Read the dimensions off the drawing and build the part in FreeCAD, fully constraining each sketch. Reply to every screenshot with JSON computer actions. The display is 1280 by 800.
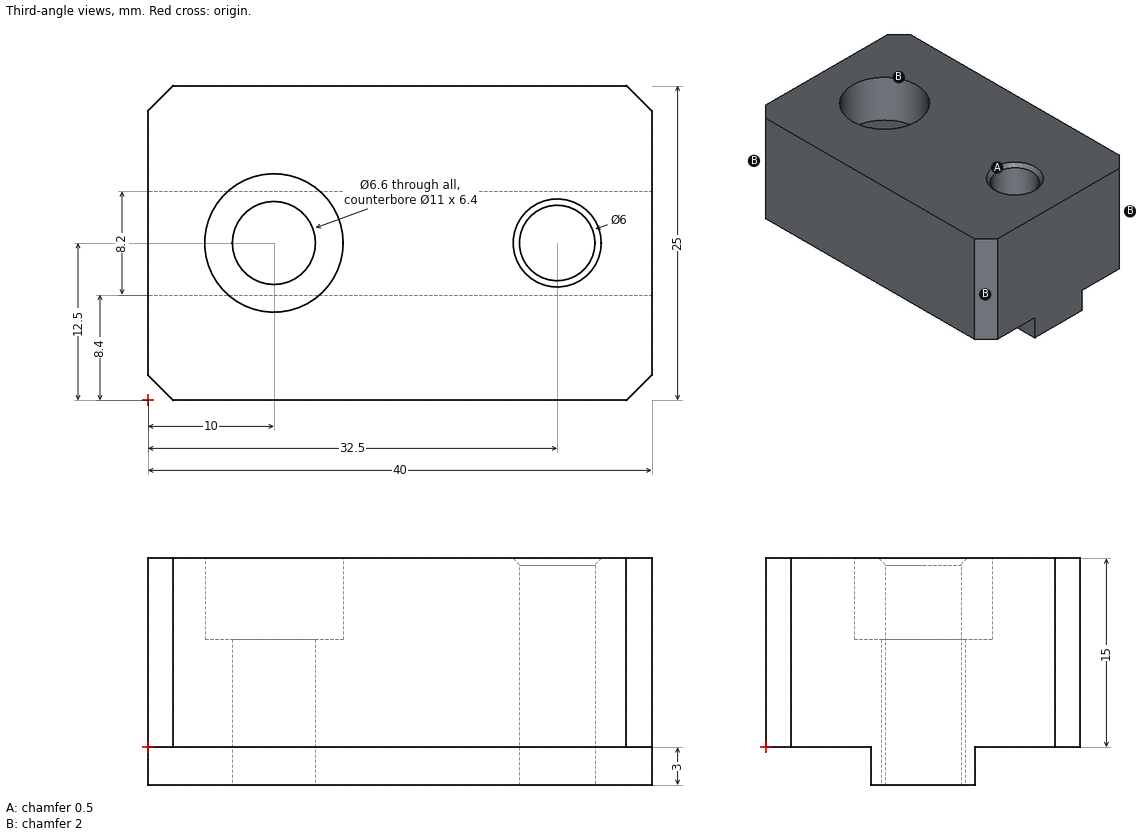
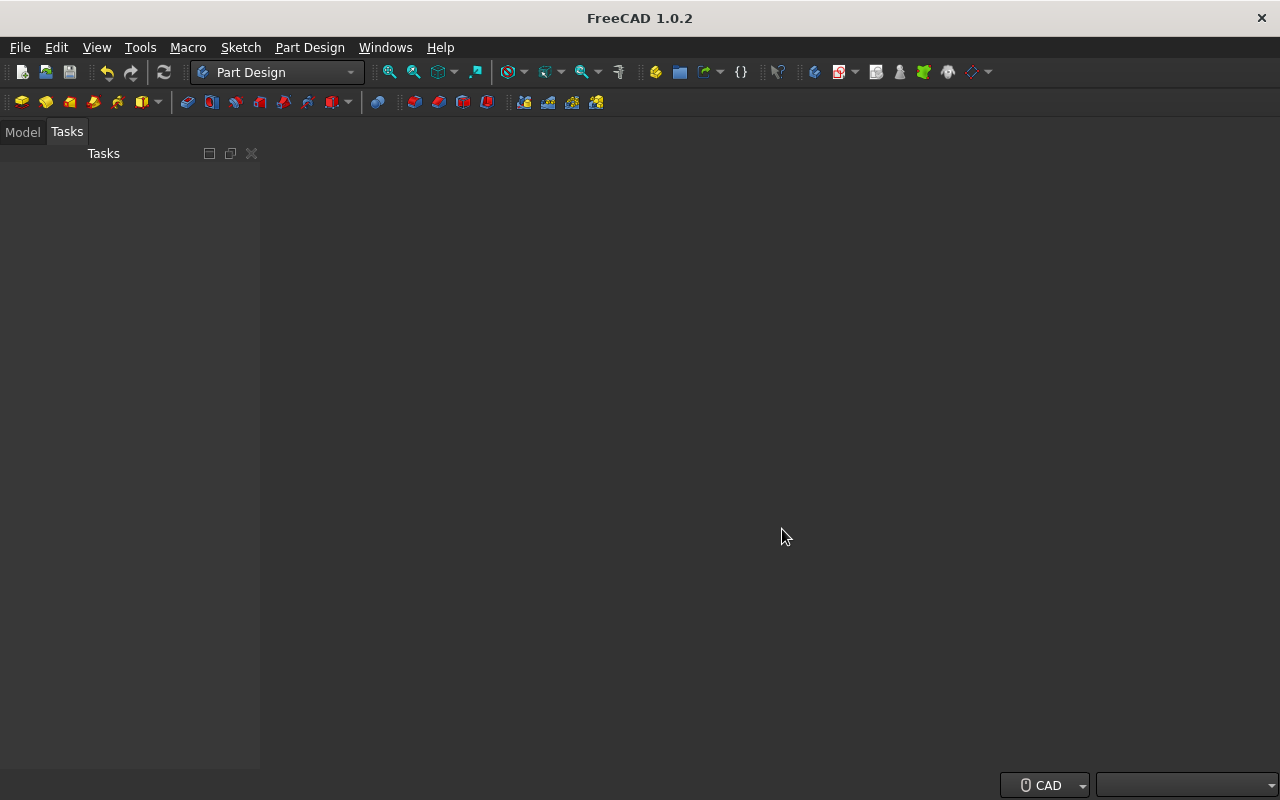
{"action": "left_click", "coordinate": [22, 72]}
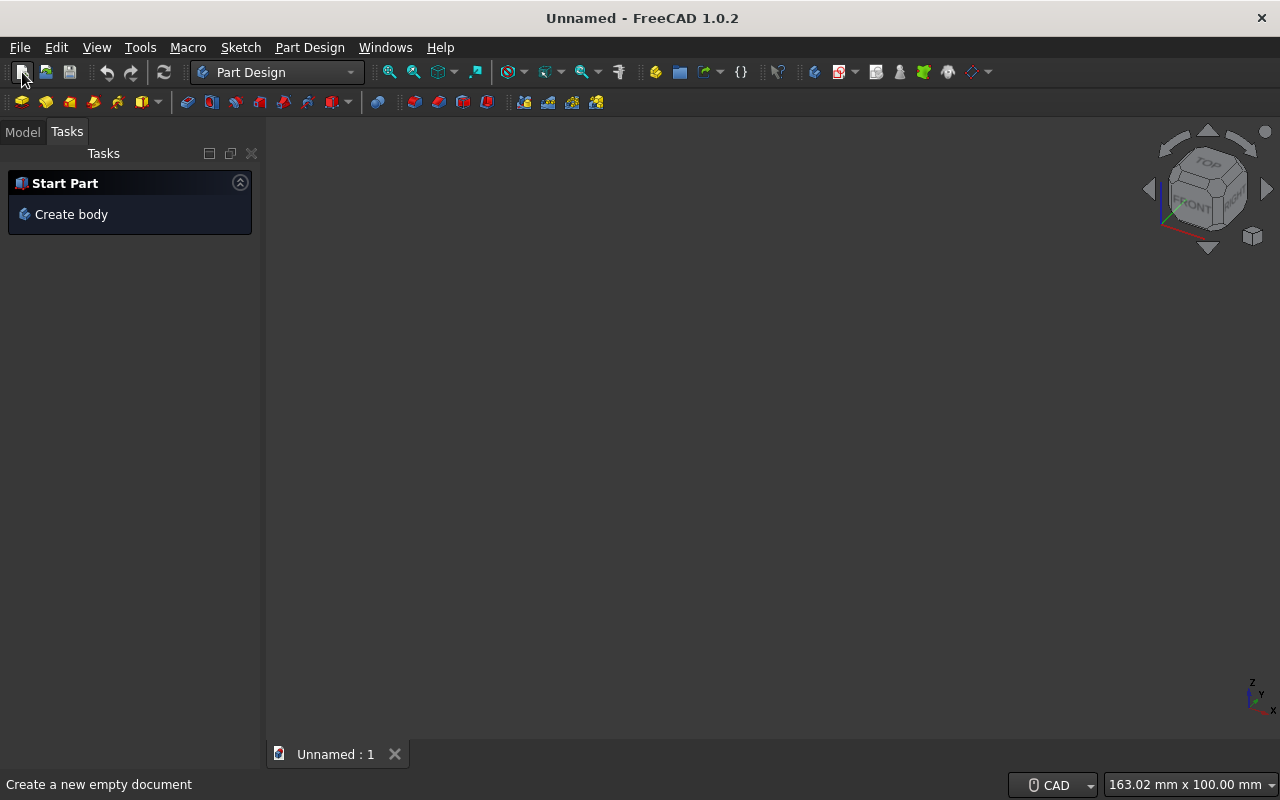
{"action": "left_click", "coordinate": [840, 72]}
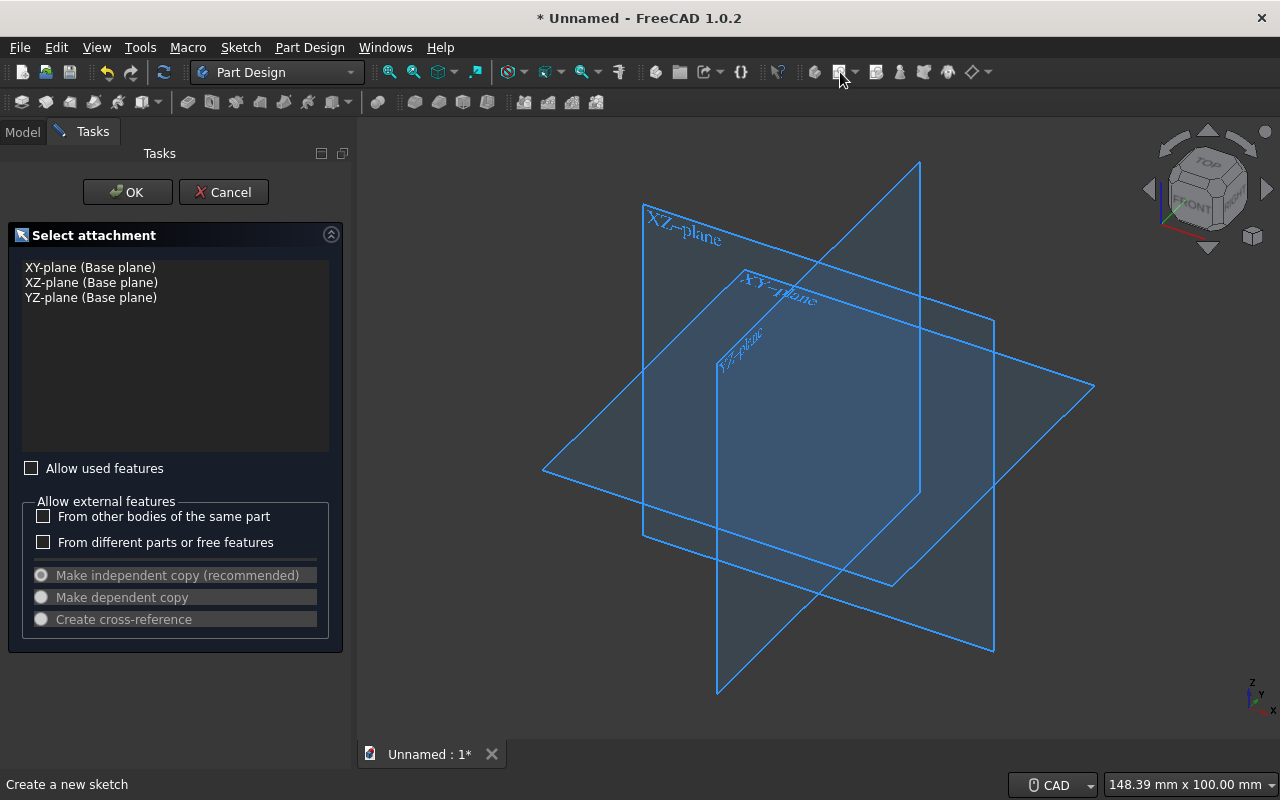
{"action": "left_click", "coordinate": [82, 268]}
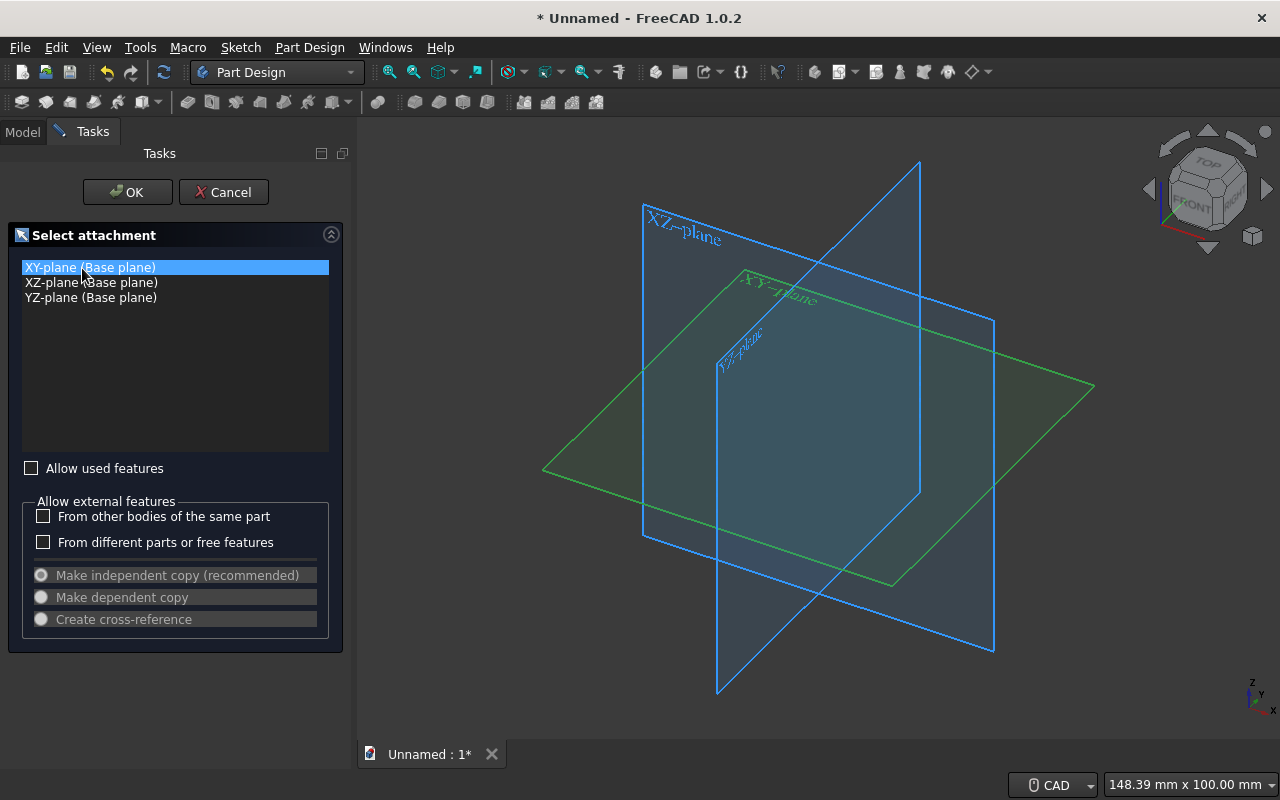
{"action": "left_click", "coordinate": [128, 192]}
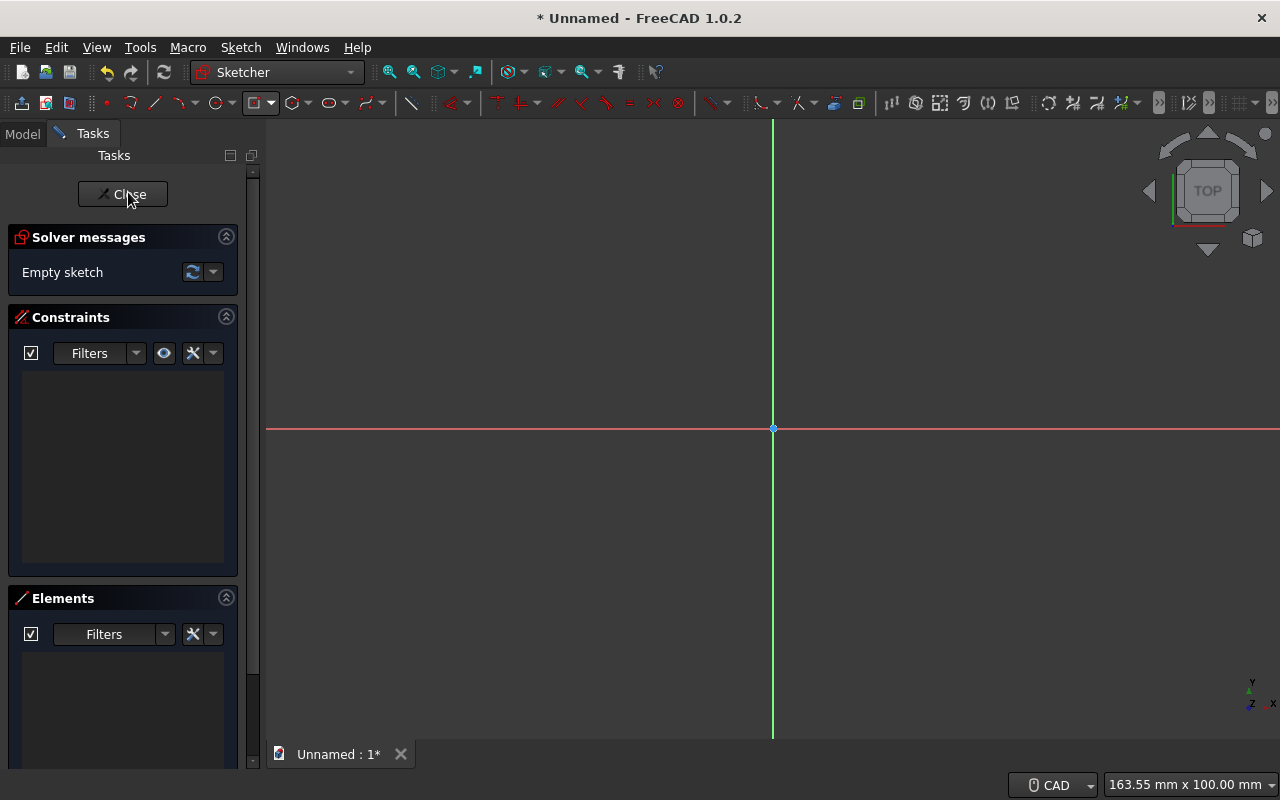
{"action": "scroll", "coordinate": [1054, 288], "scroll_direction": "up", "scroll_amount": 4}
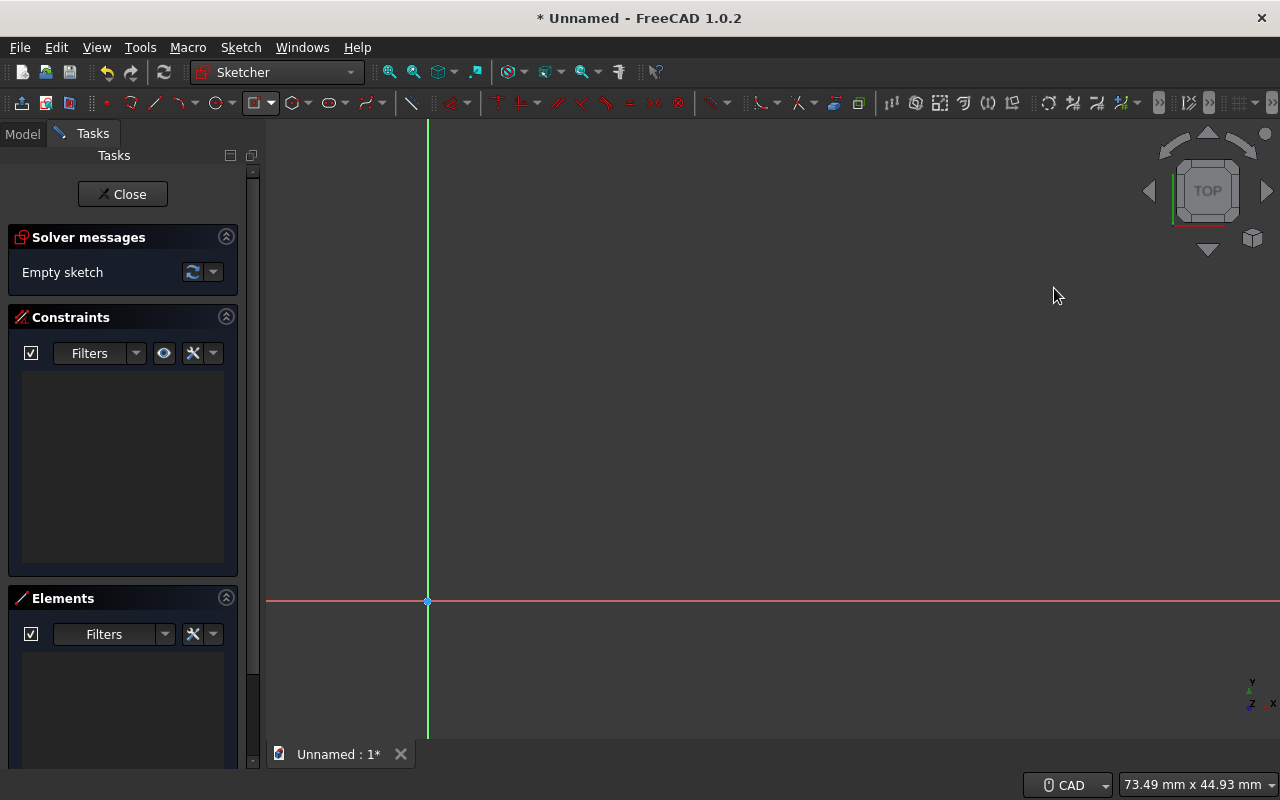
{"action": "key", "text": "g r"}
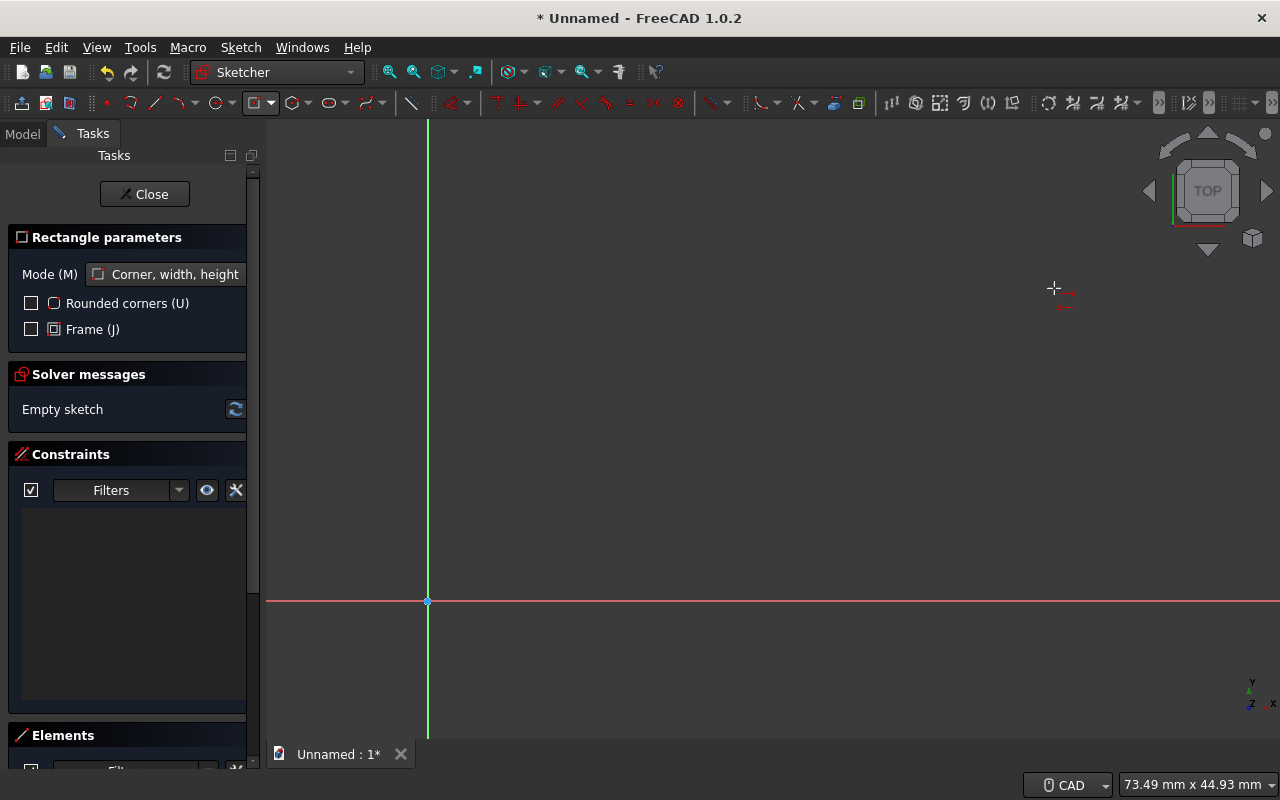
{"action": "left_click", "coordinate": [428, 601]}
{"action": "left_click", "coordinate": [980, 257]}
{"action": "key", "text": "Escape"}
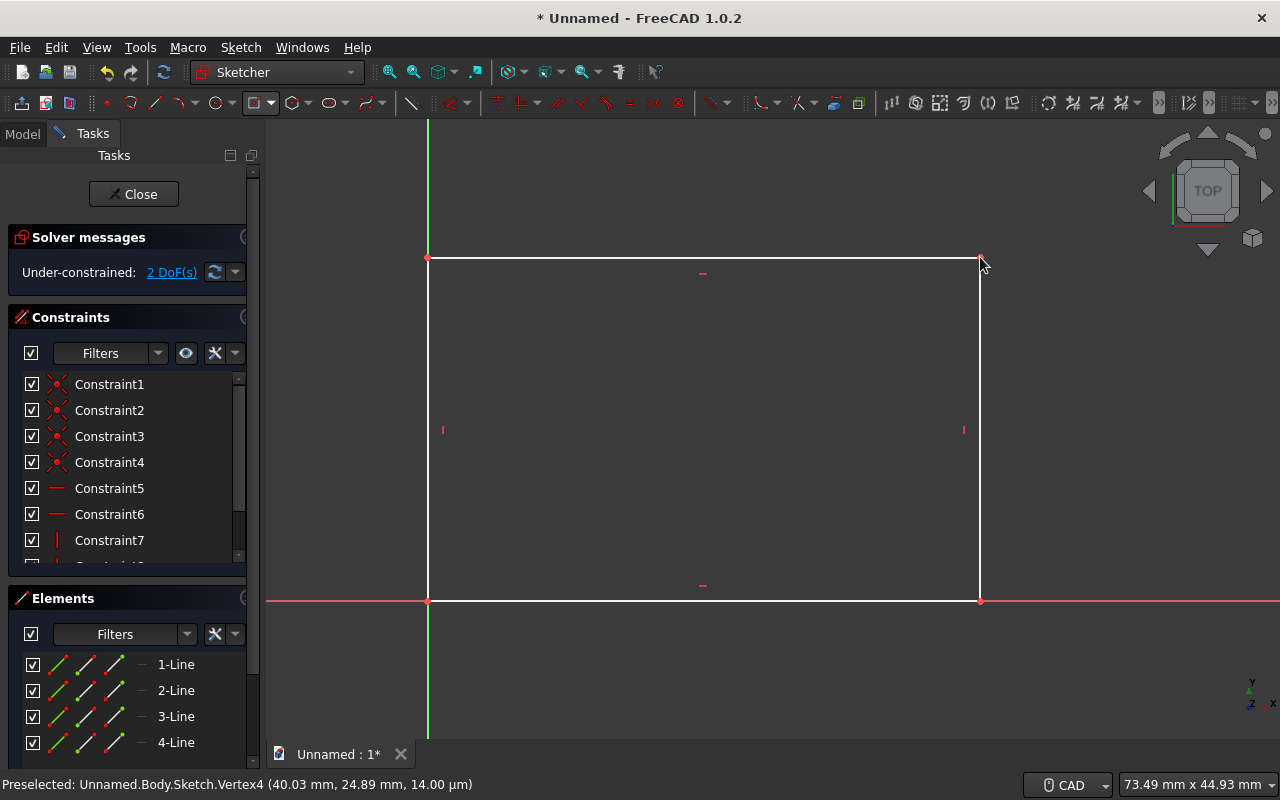
{"action": "left_click", "coordinate": [450, 104]}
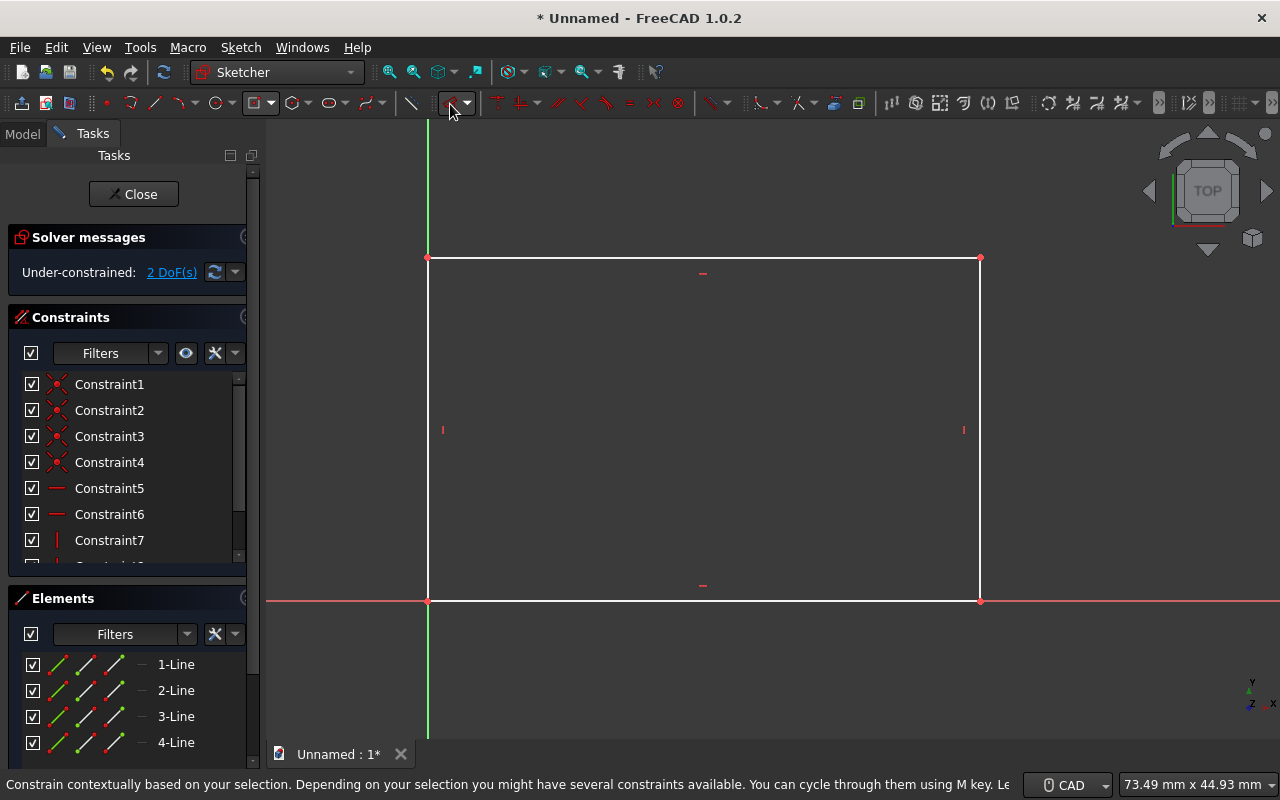
{"action": "left_click", "coordinate": [593, 601]}
{"action": "left_click", "coordinate": [704, 635]}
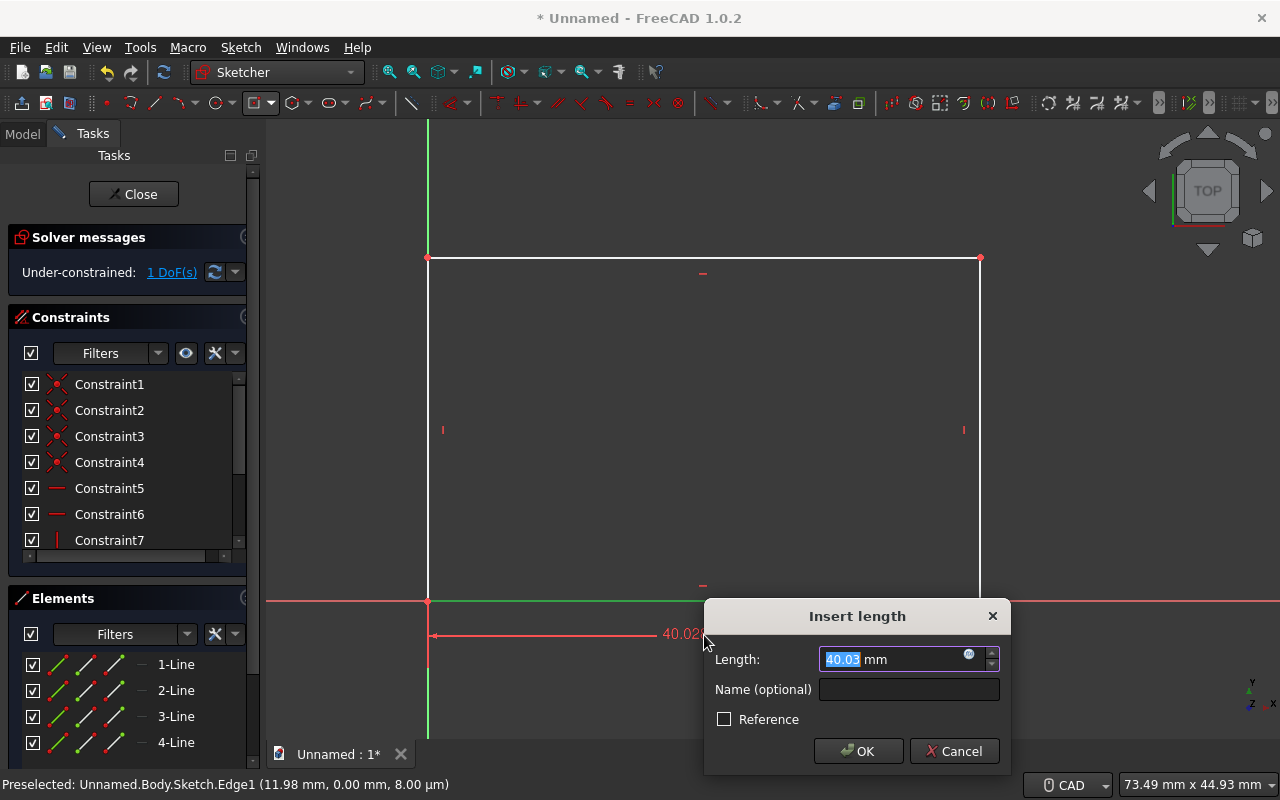
{"action": "type", "text": "40"}
{"action": "key", "text": "Return"}